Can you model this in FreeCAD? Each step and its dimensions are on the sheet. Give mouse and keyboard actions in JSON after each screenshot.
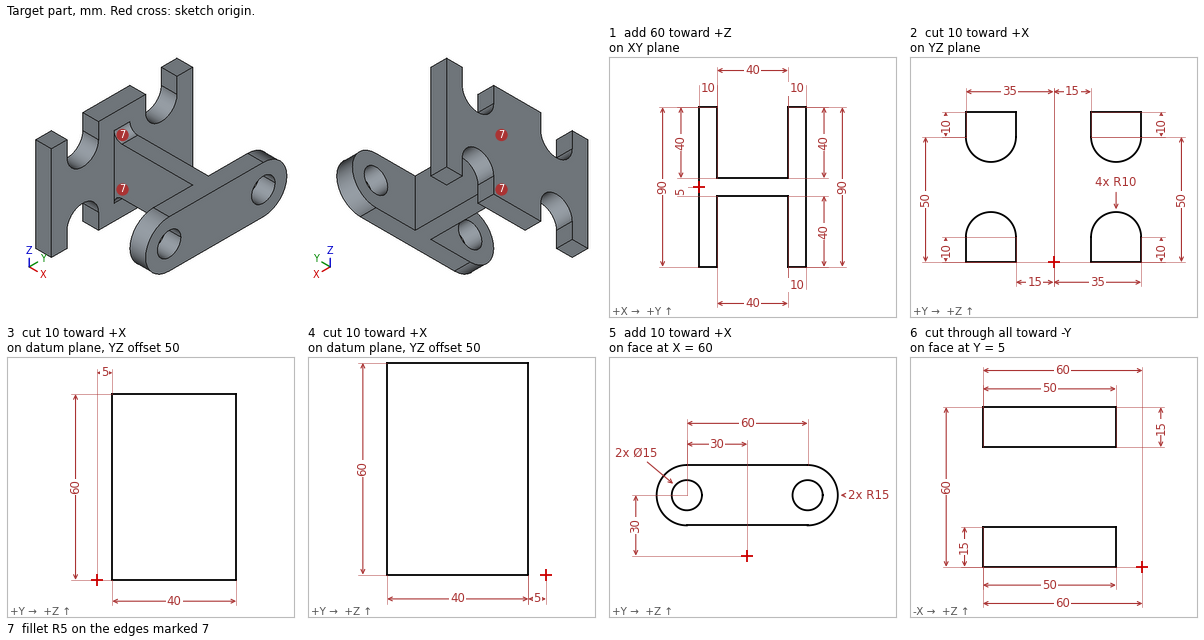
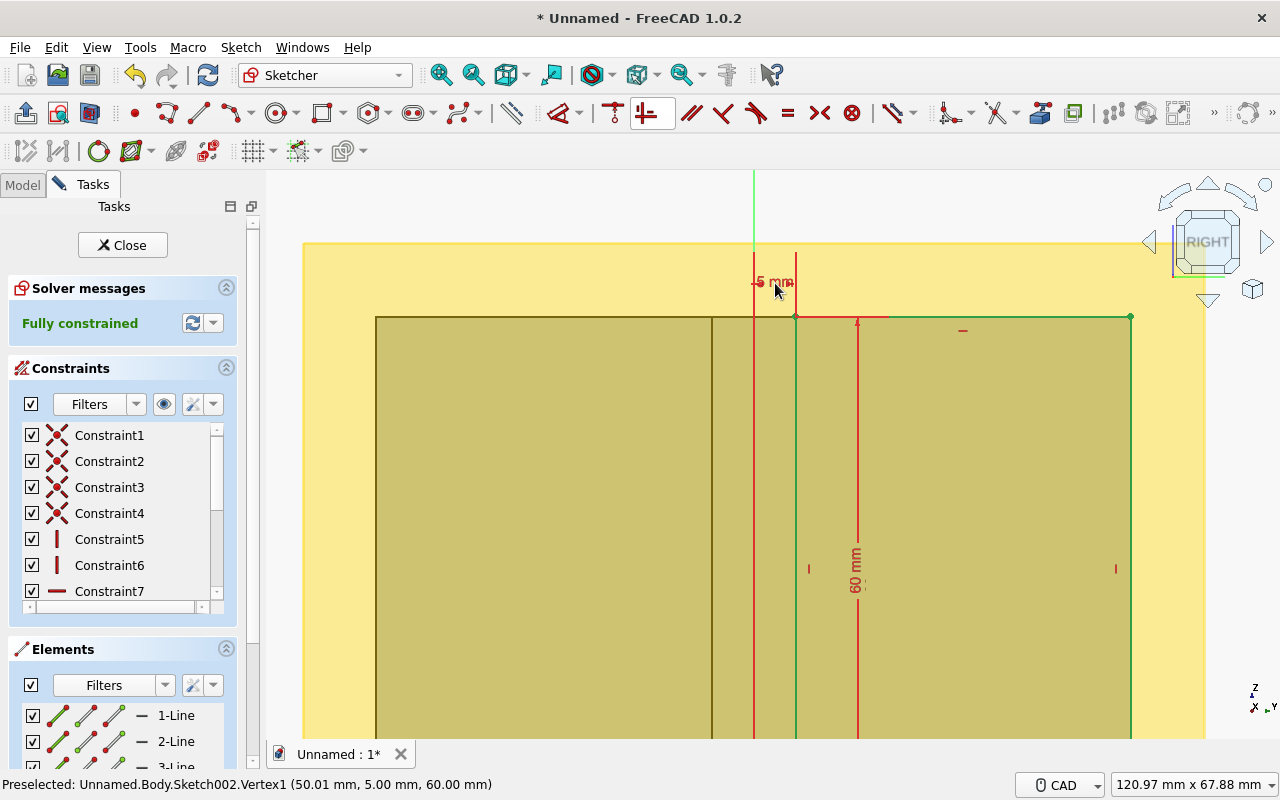
{"action": "left_click", "coordinate": [123, 245]}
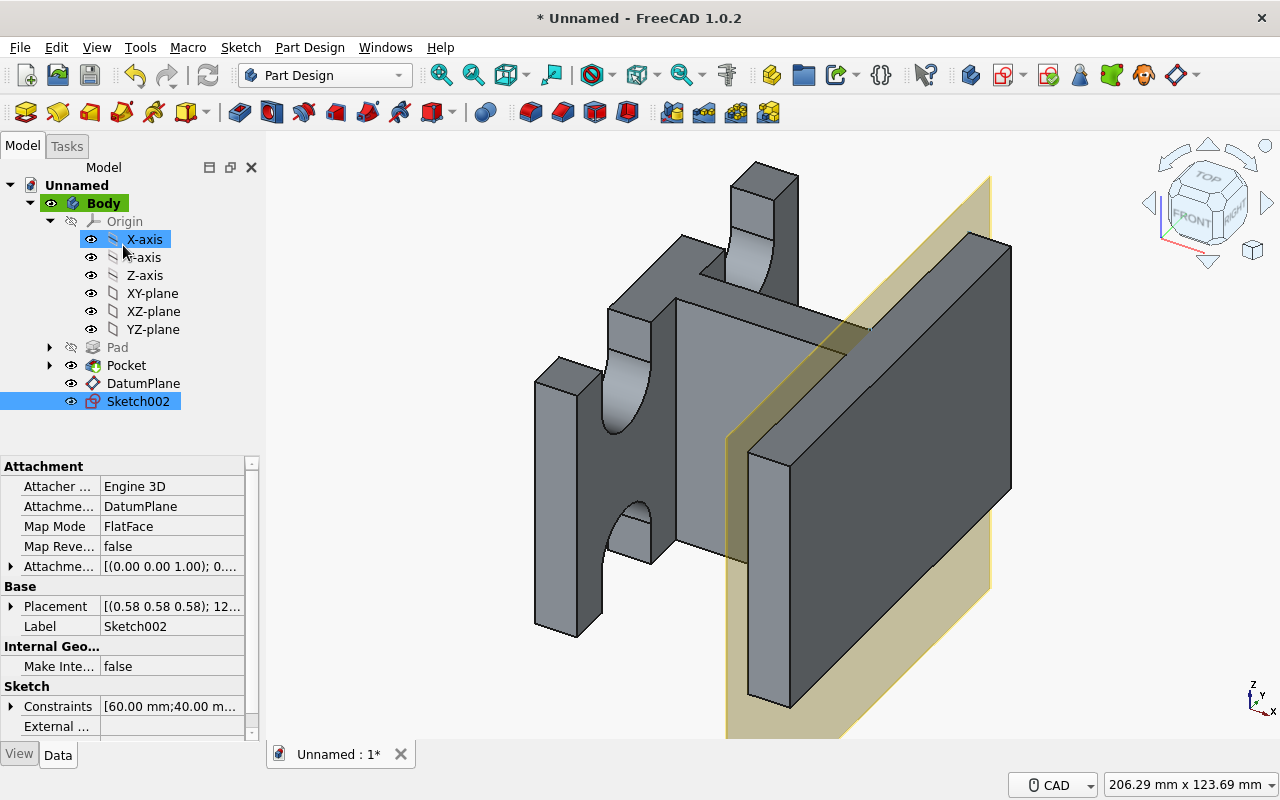
{"action": "left_click", "coordinate": [240, 112]}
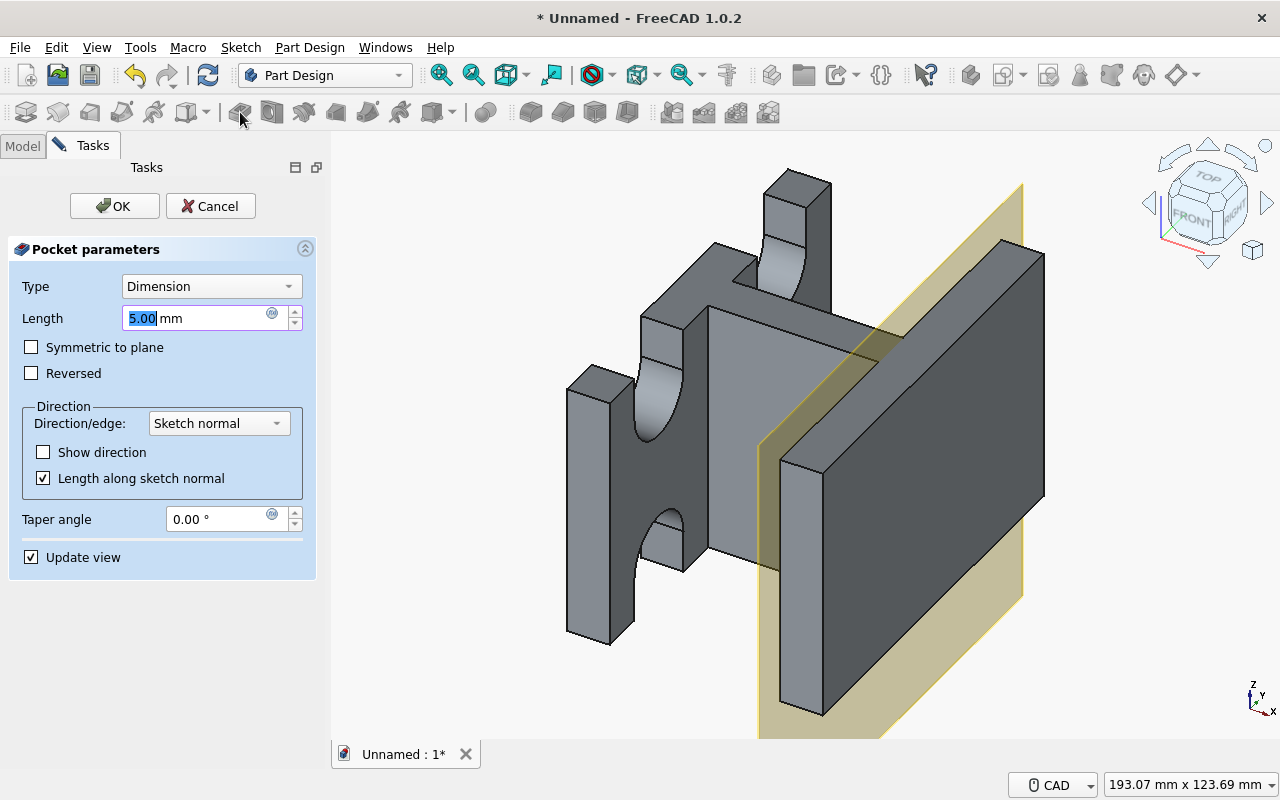
{"action": "type", "text": "10"}
{"action": "key", "text": "Tab"}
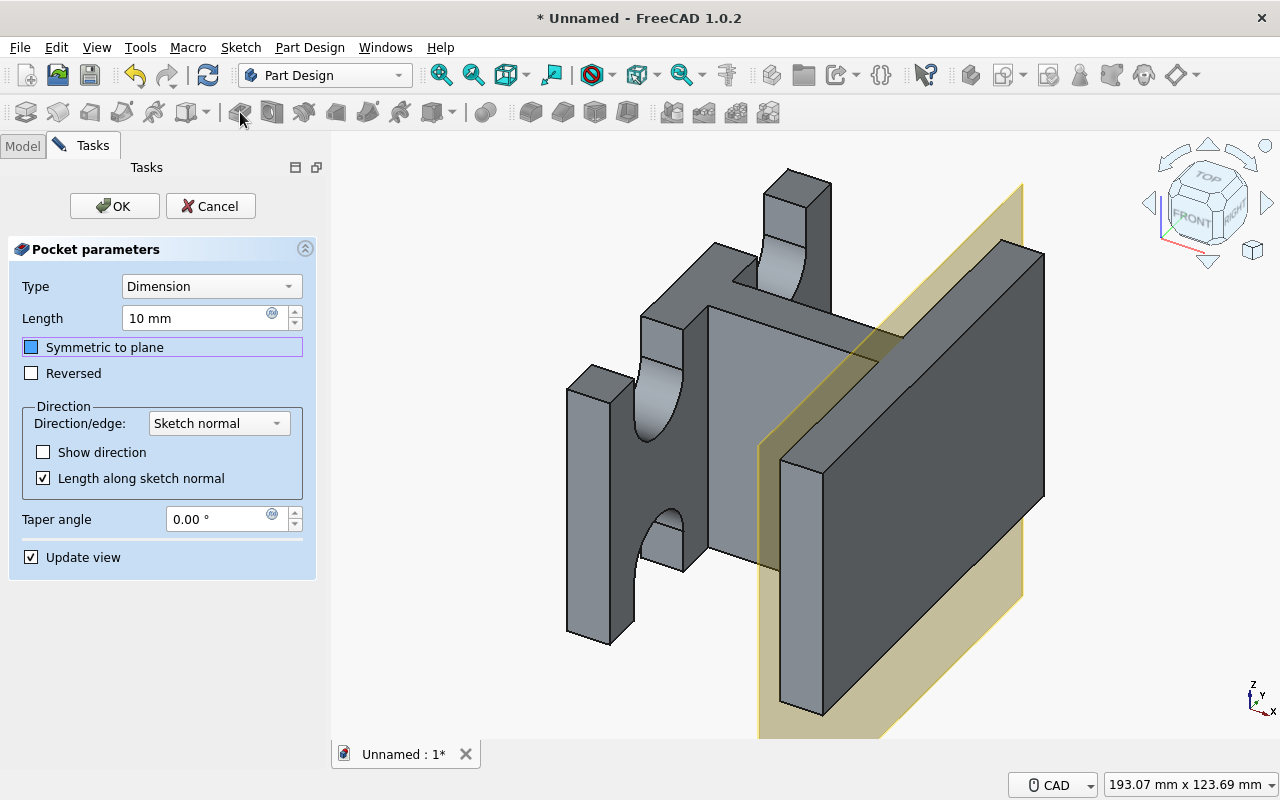
{"action": "left_click", "coordinate": [30, 373]}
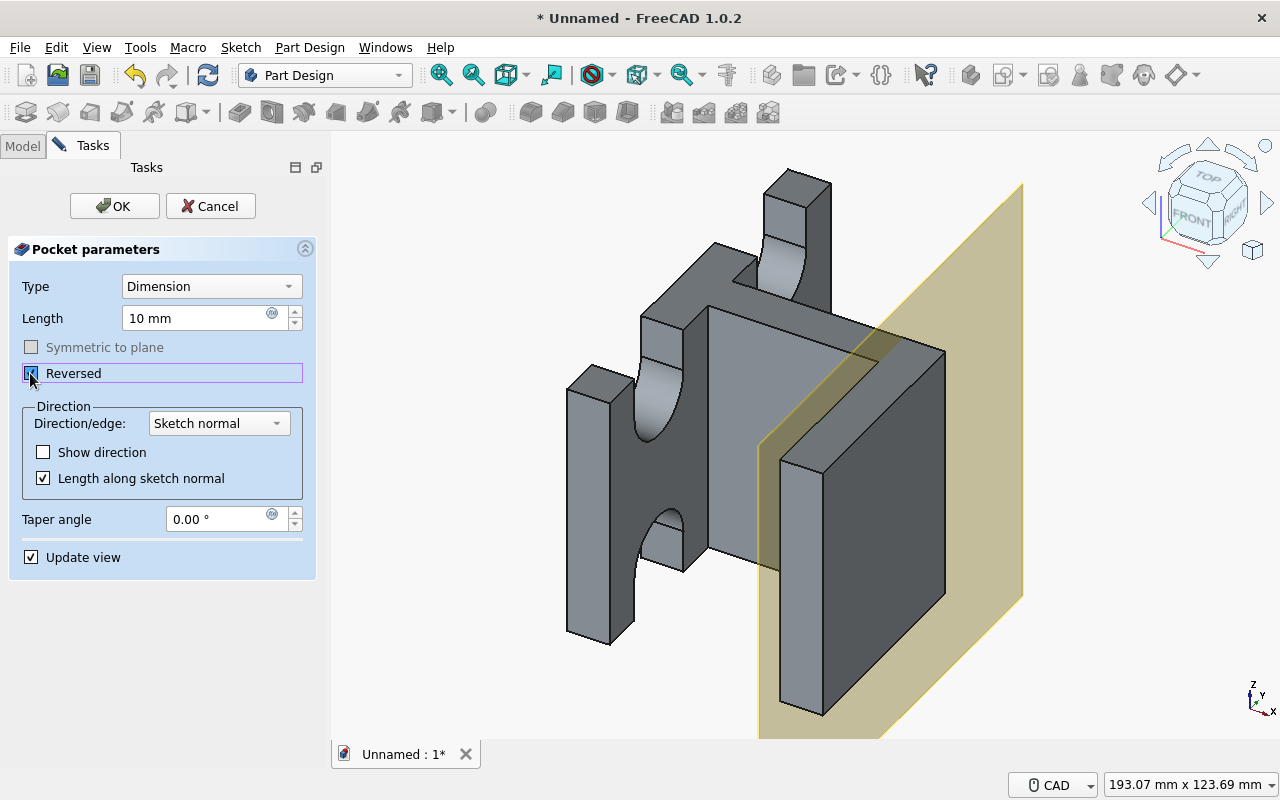
{"action": "left_click", "coordinate": [115, 206]}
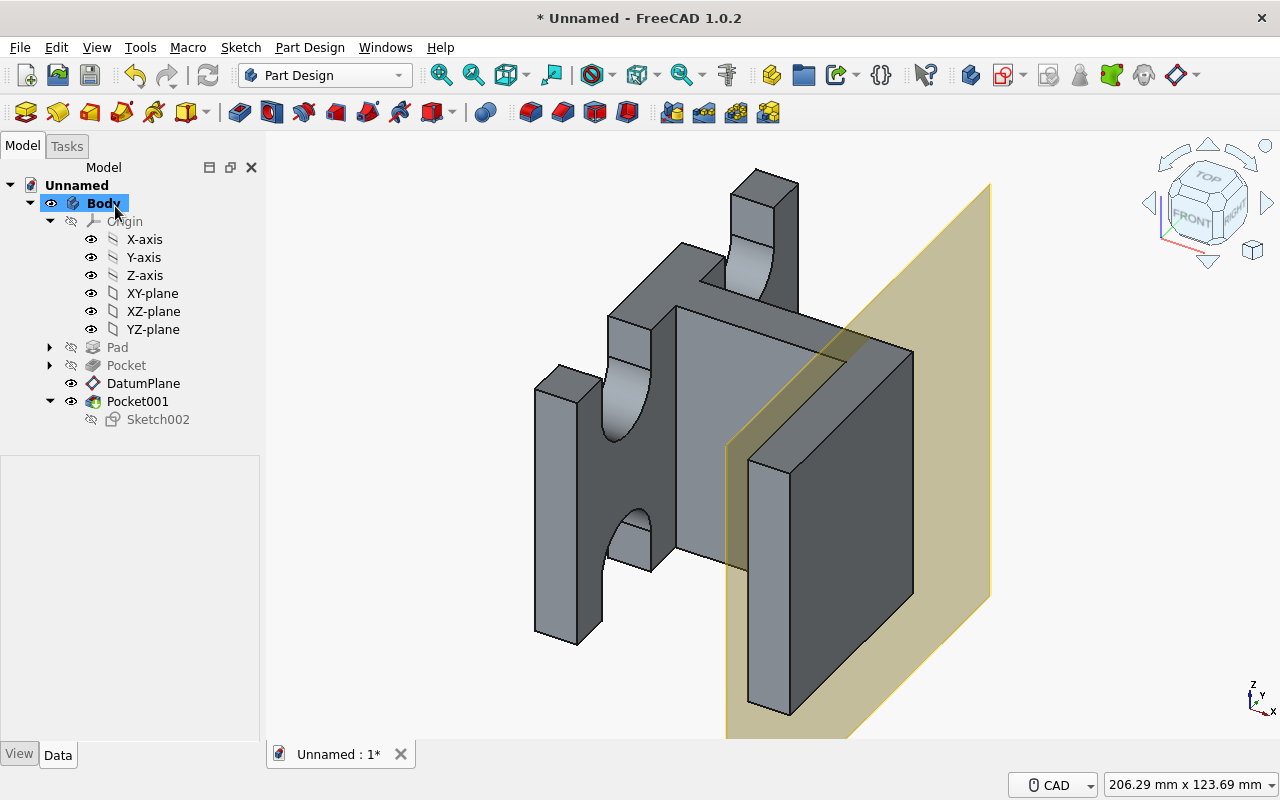
{"action": "left_click", "coordinate": [116, 383]}
{"action": "key", "text": "space"}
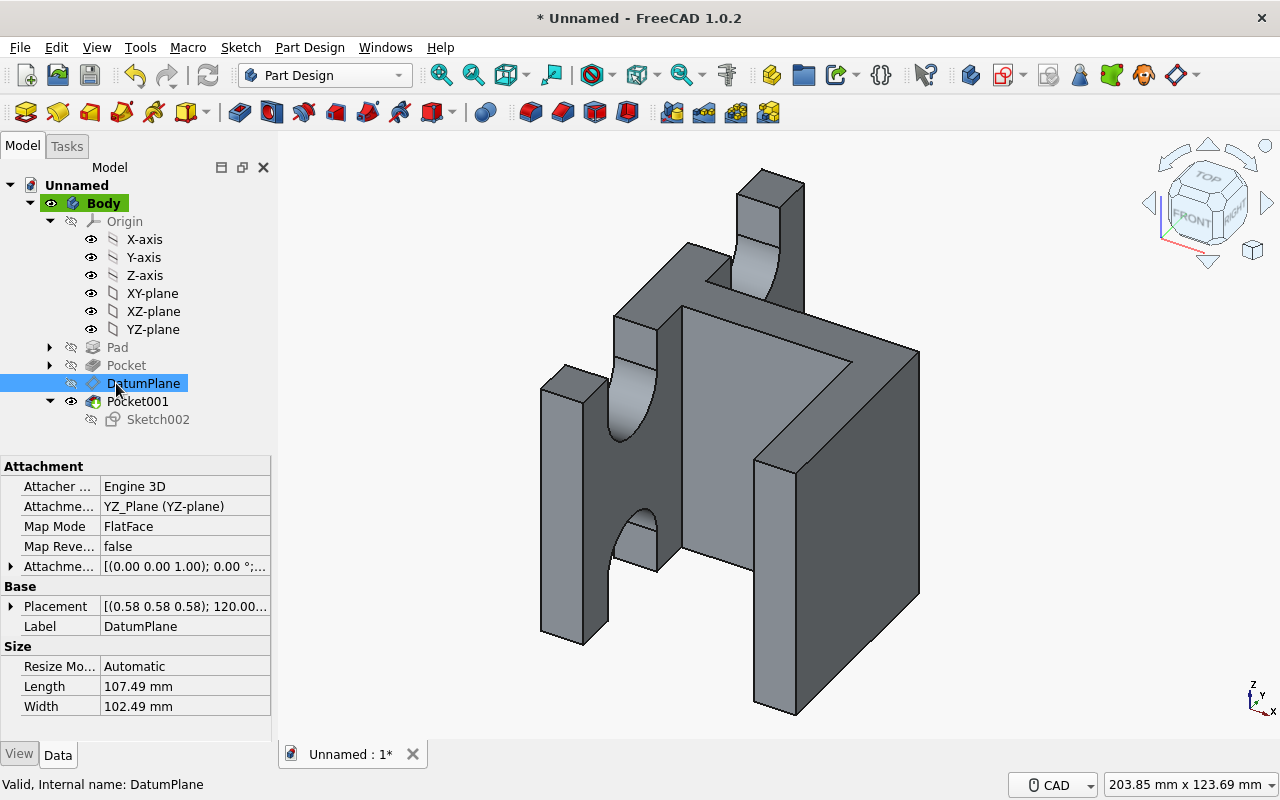
{"action": "left_click", "coordinate": [136, 329]}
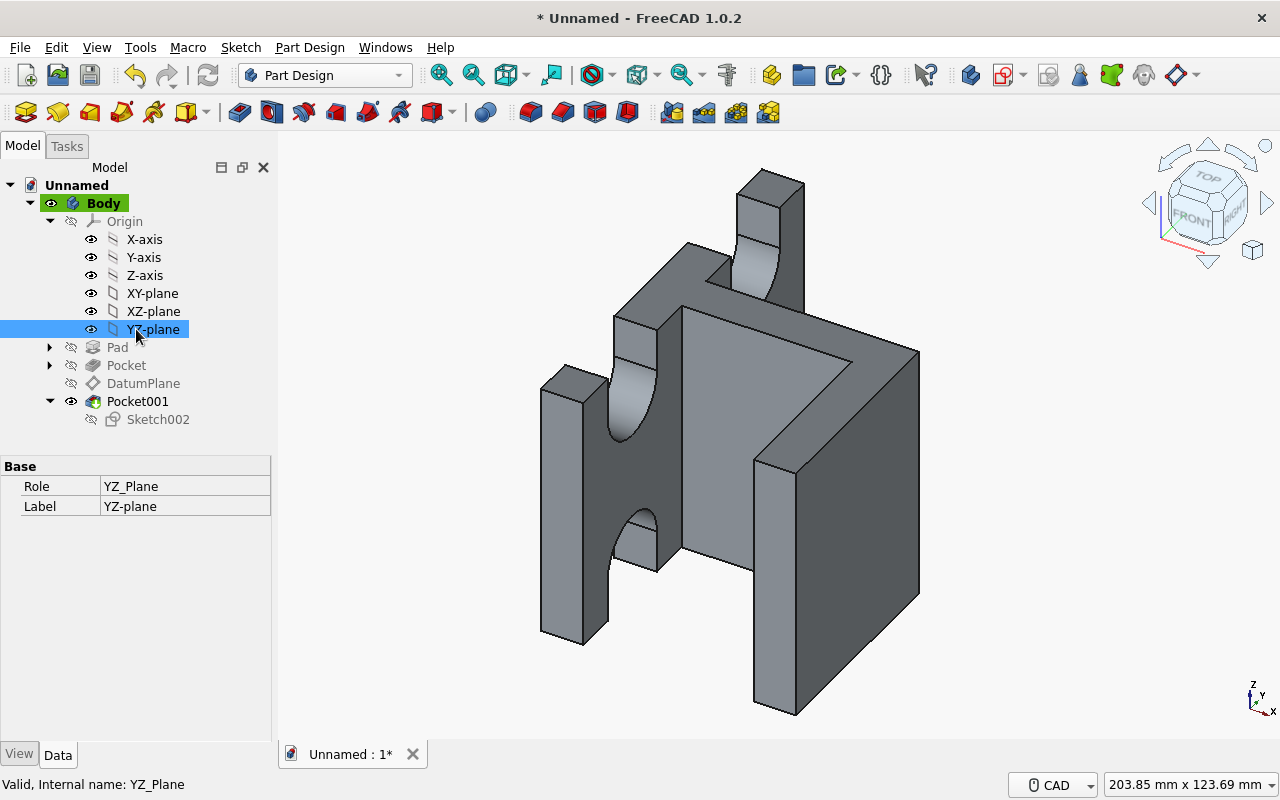
{"action": "left_click", "coordinate": [1176, 76]}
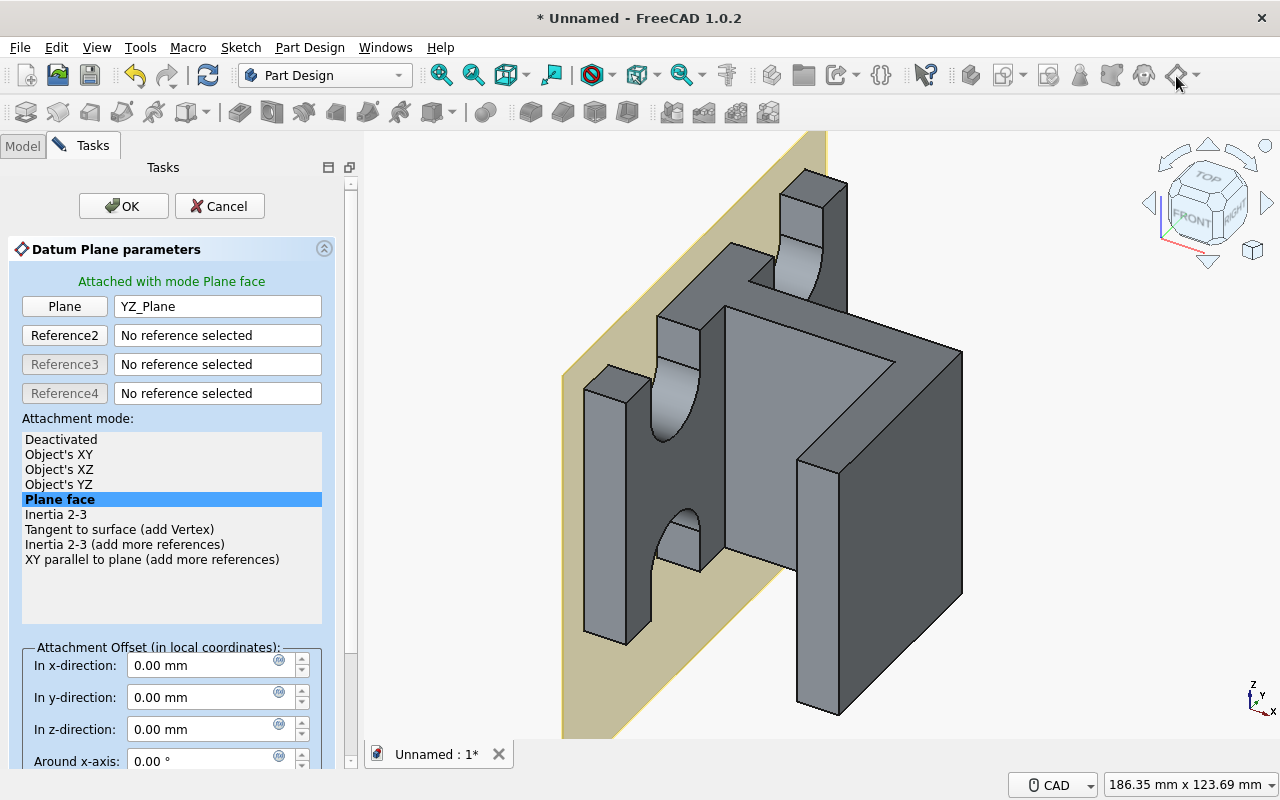
{"action": "triple_click", "coordinate": [210, 729]}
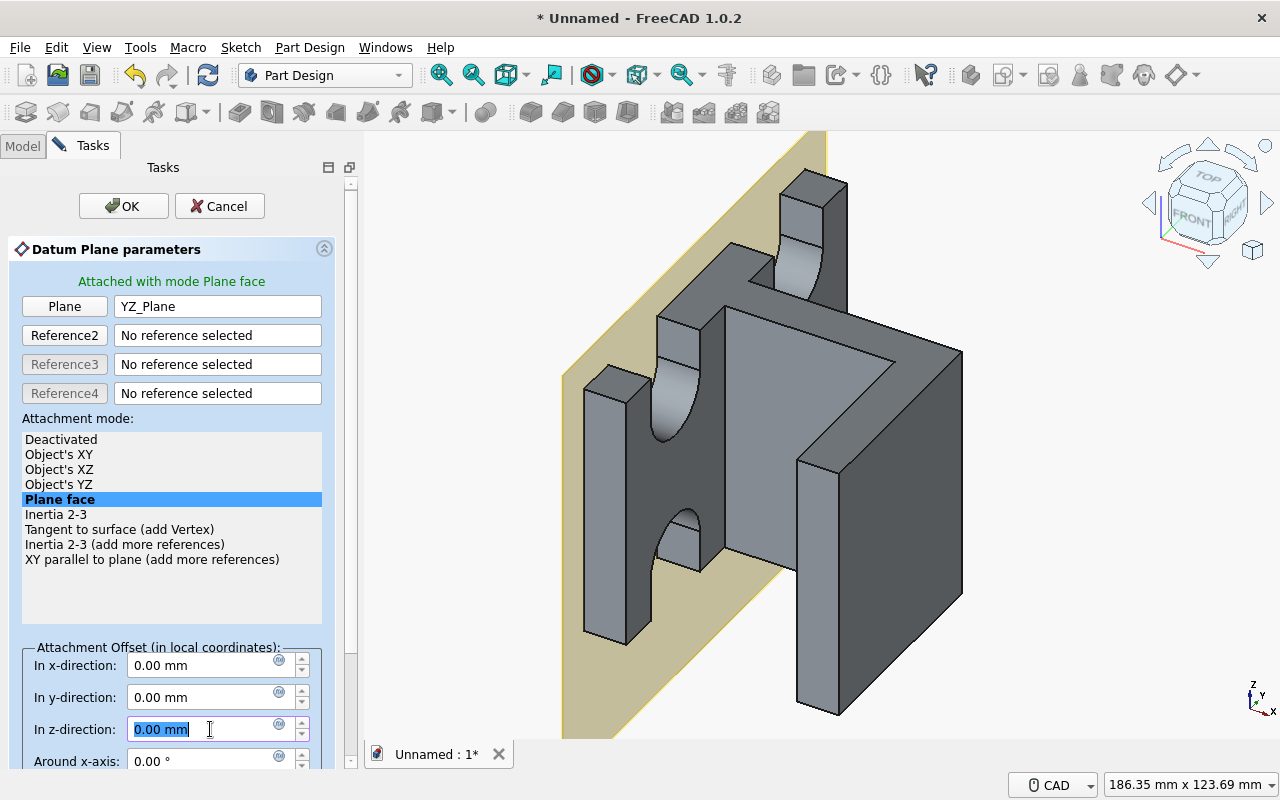
{"action": "type", "text": "50"}
{"action": "key", "text": "Tab"}